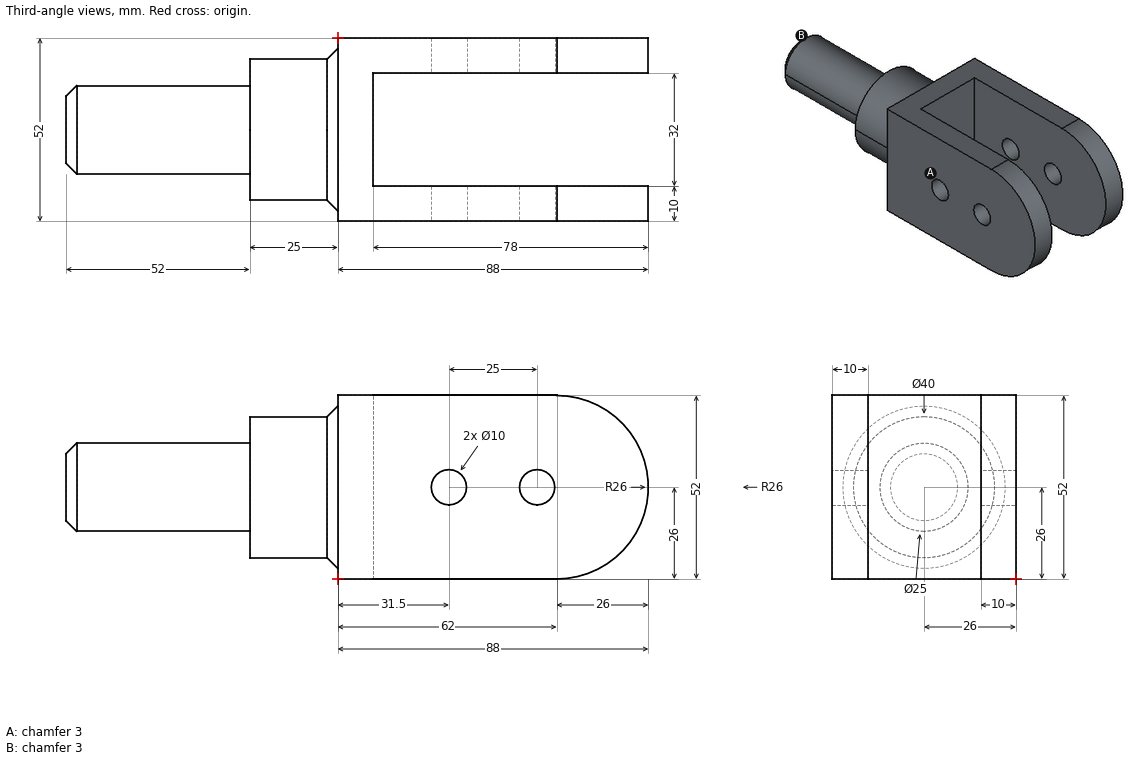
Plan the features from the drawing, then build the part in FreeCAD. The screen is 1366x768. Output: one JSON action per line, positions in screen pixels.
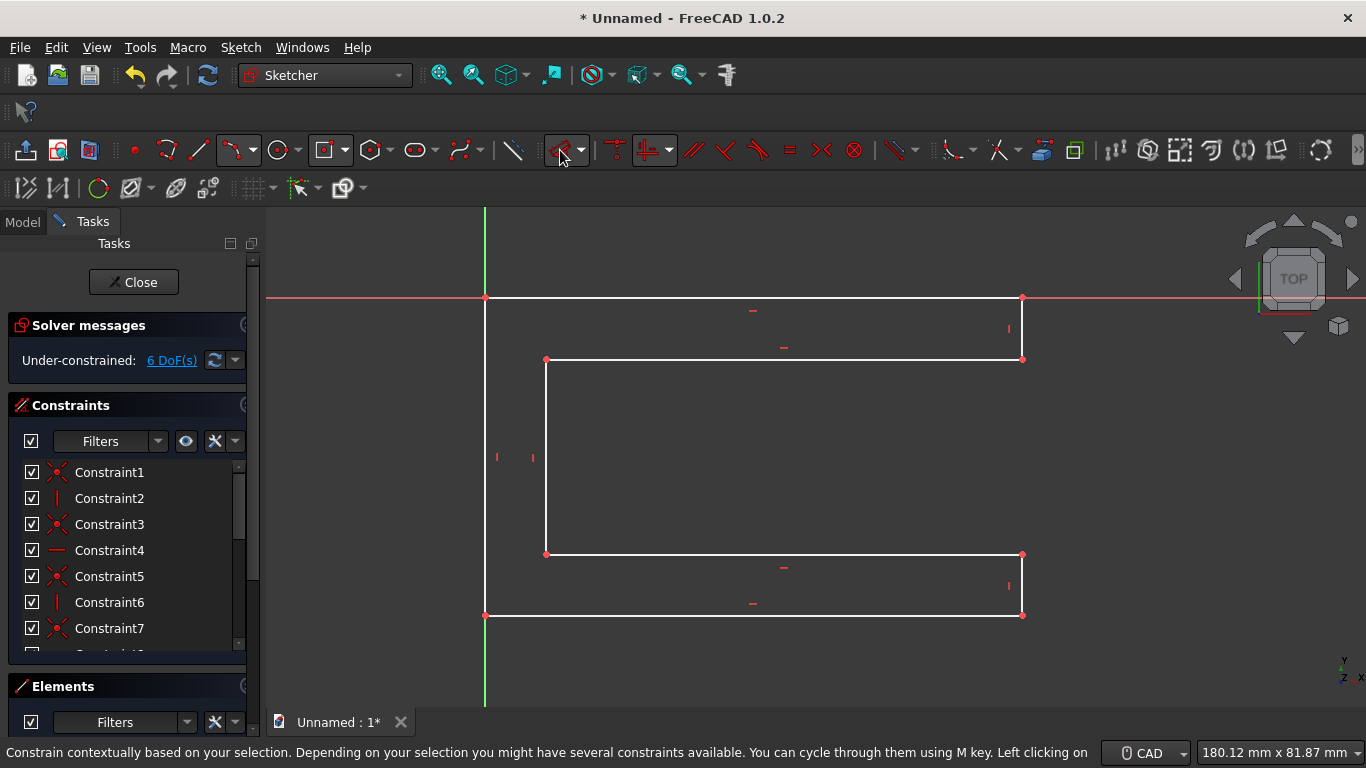
{"action": "left_click", "coordinate": [485, 393]}
{"action": "left_click", "coordinate": [451, 457]}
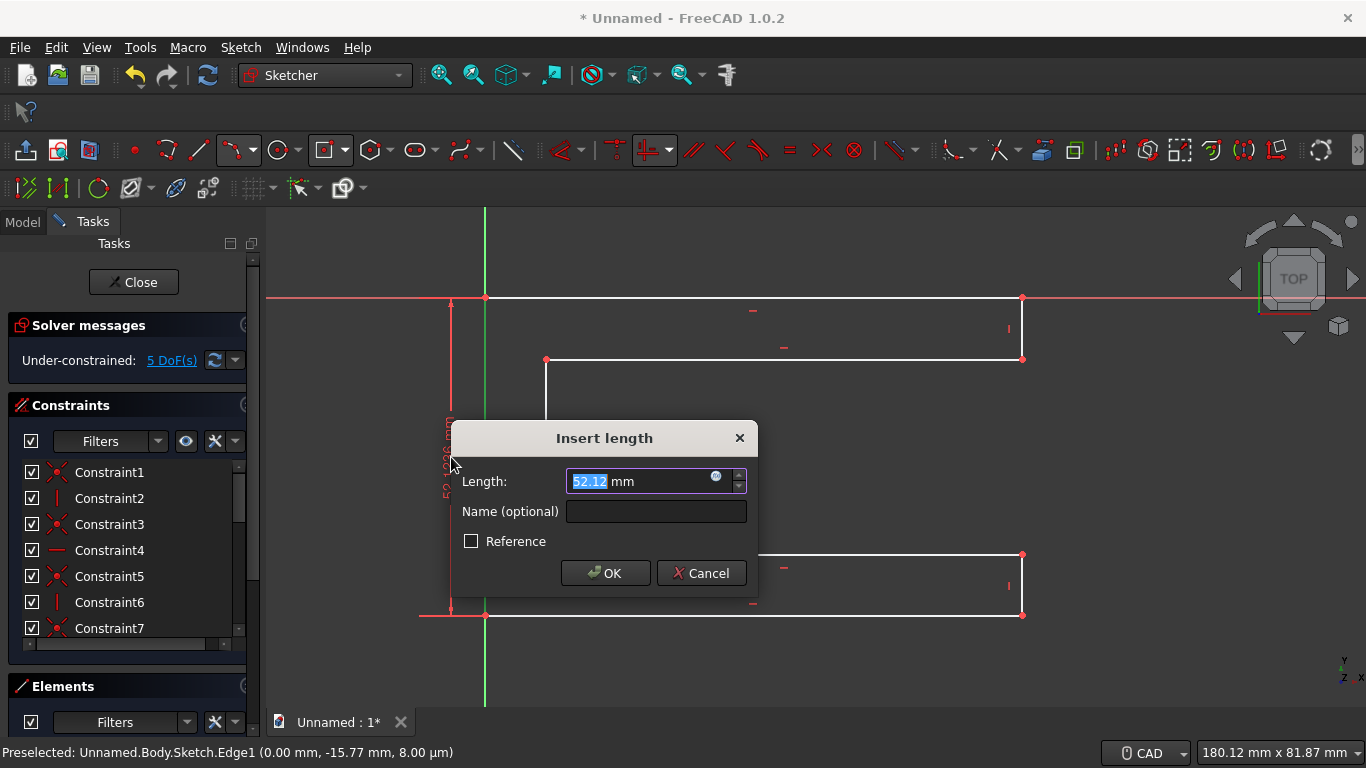
{"action": "type", "text": "52"}
{"action": "key", "text": "Return"}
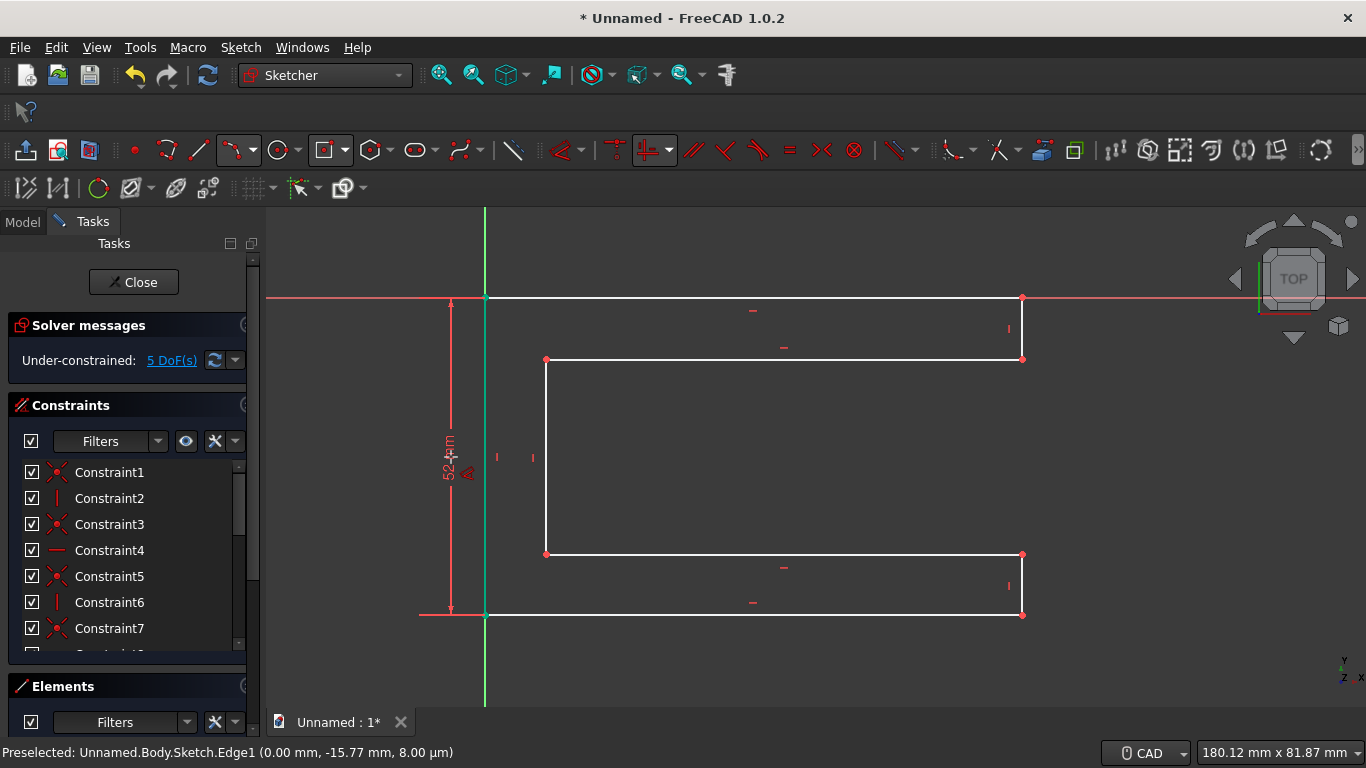
{"action": "left_click", "coordinate": [646, 615]}
{"action": "left_click", "coordinate": [754, 649]}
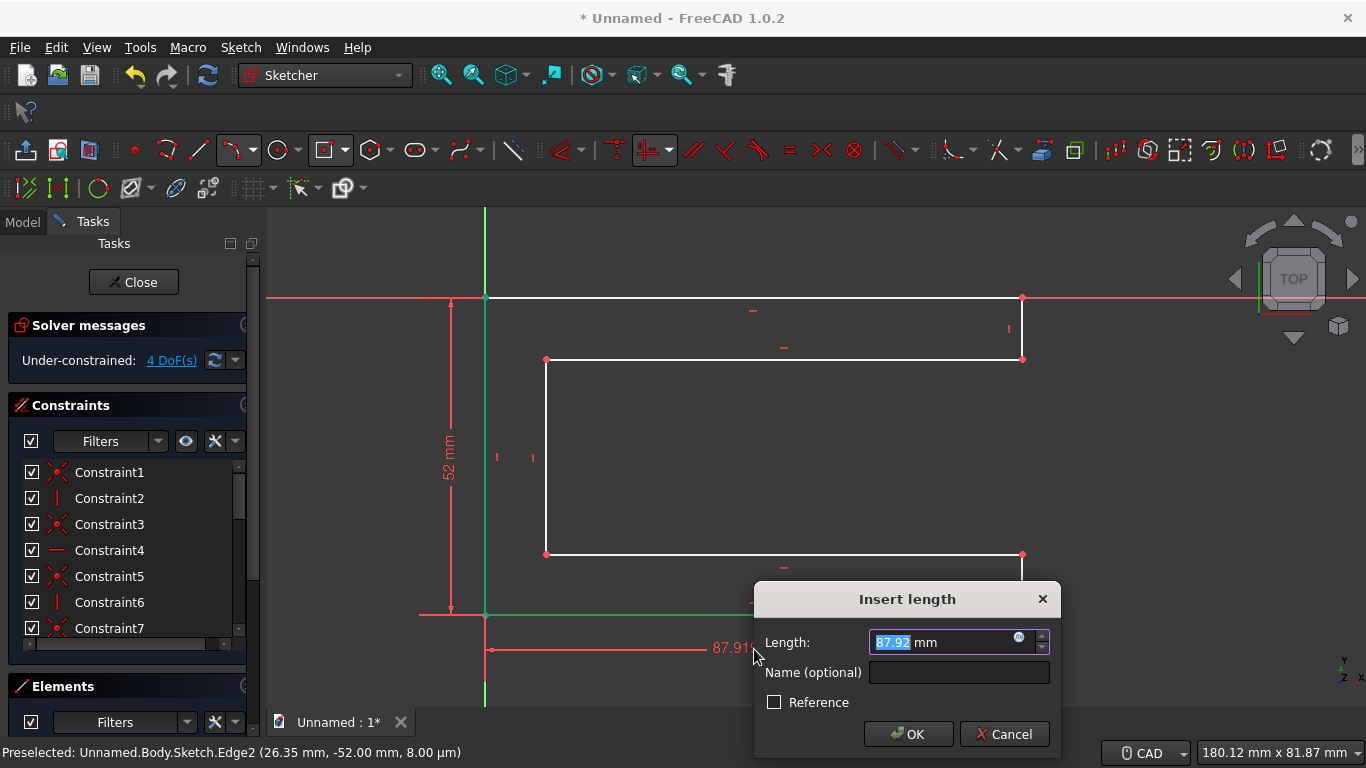
{"action": "type", "text": "88"}
{"action": "key", "text": "Return"}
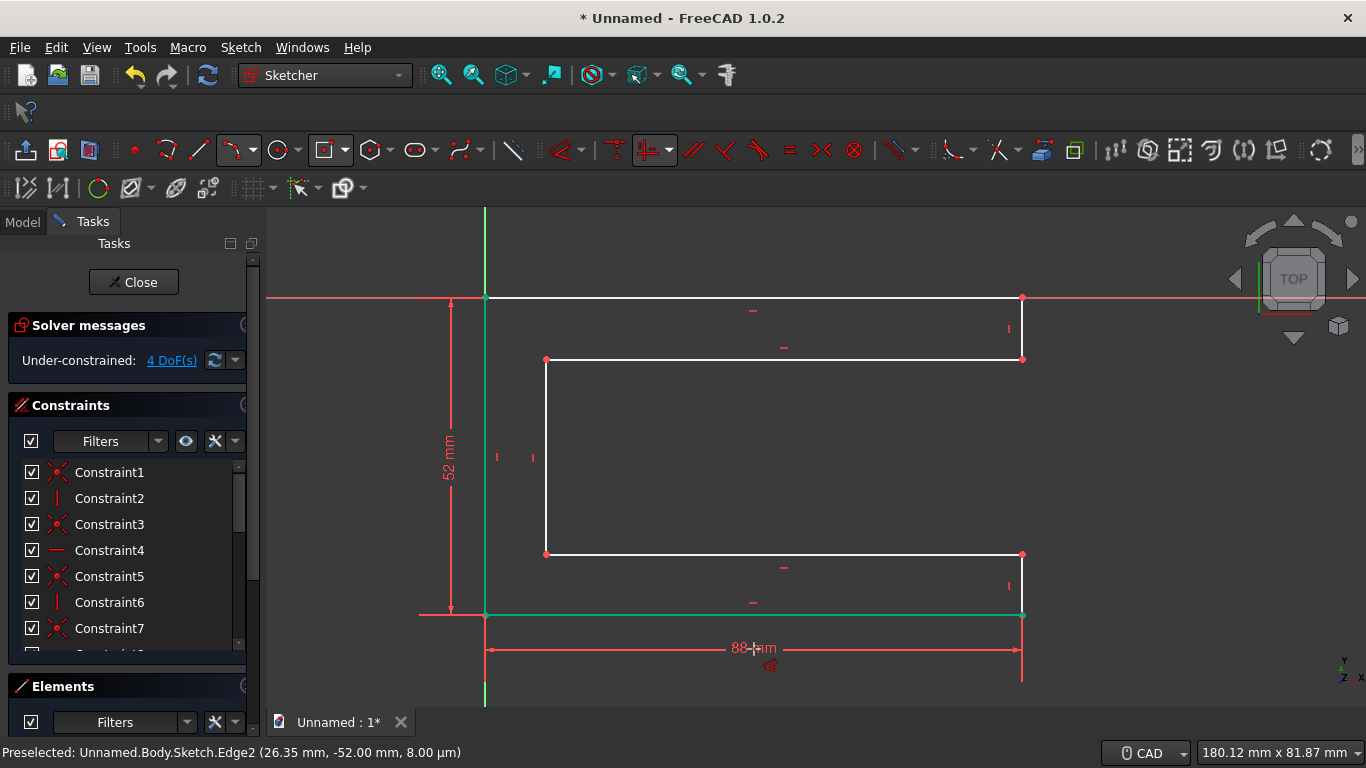
{"action": "left_click", "coordinate": [1022, 597]}
{"action": "left_click", "coordinate": [1056, 585]}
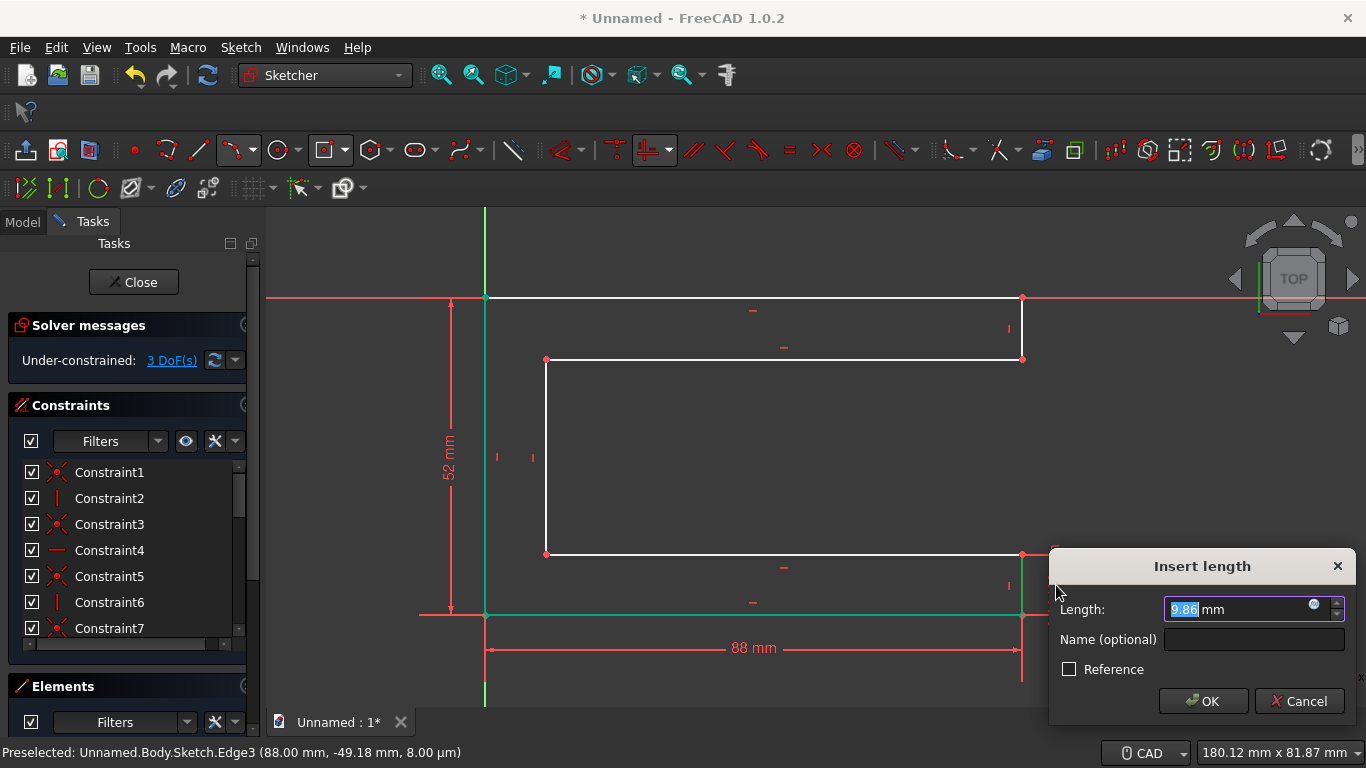
{"action": "type", "text": "10"}
{"action": "key", "text": "Return"}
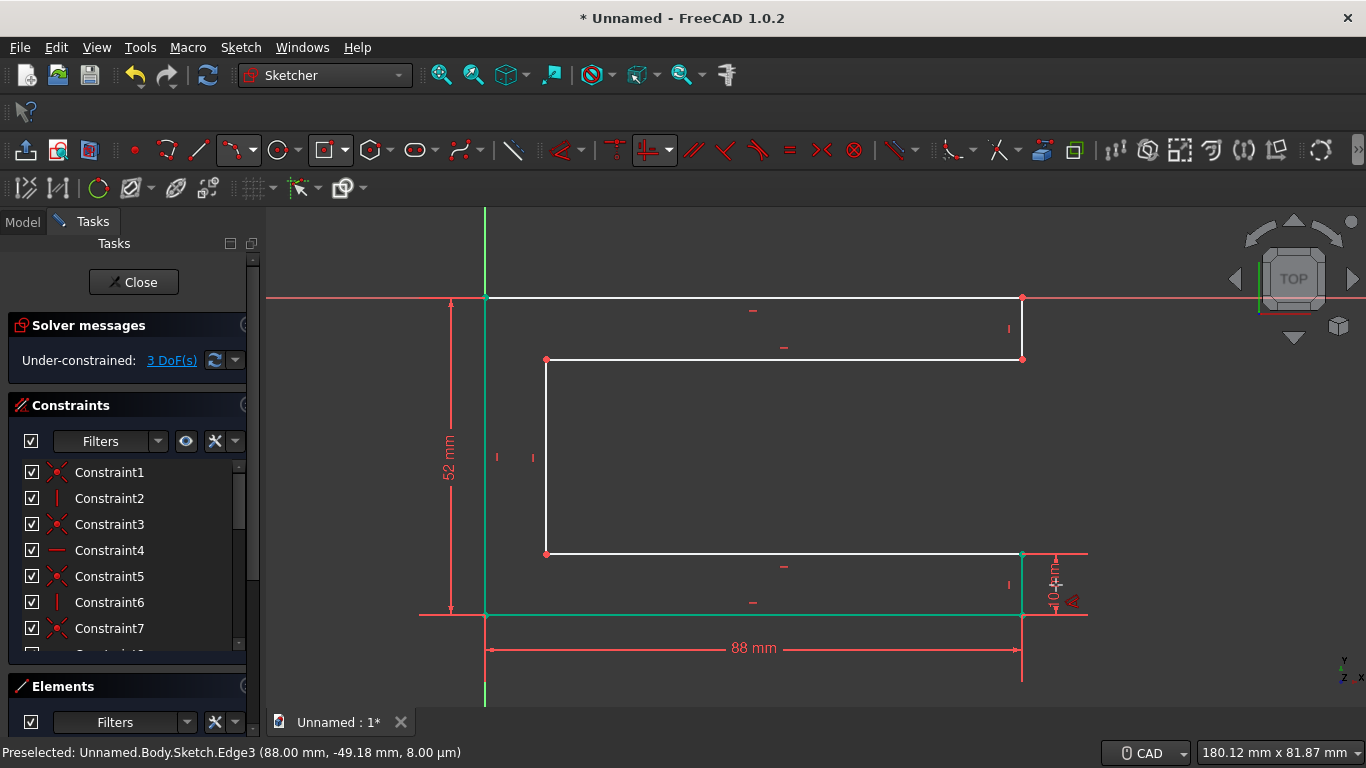
{"action": "left_click", "coordinate": [880, 554]}
{"action": "left_click", "coordinate": [784, 588]}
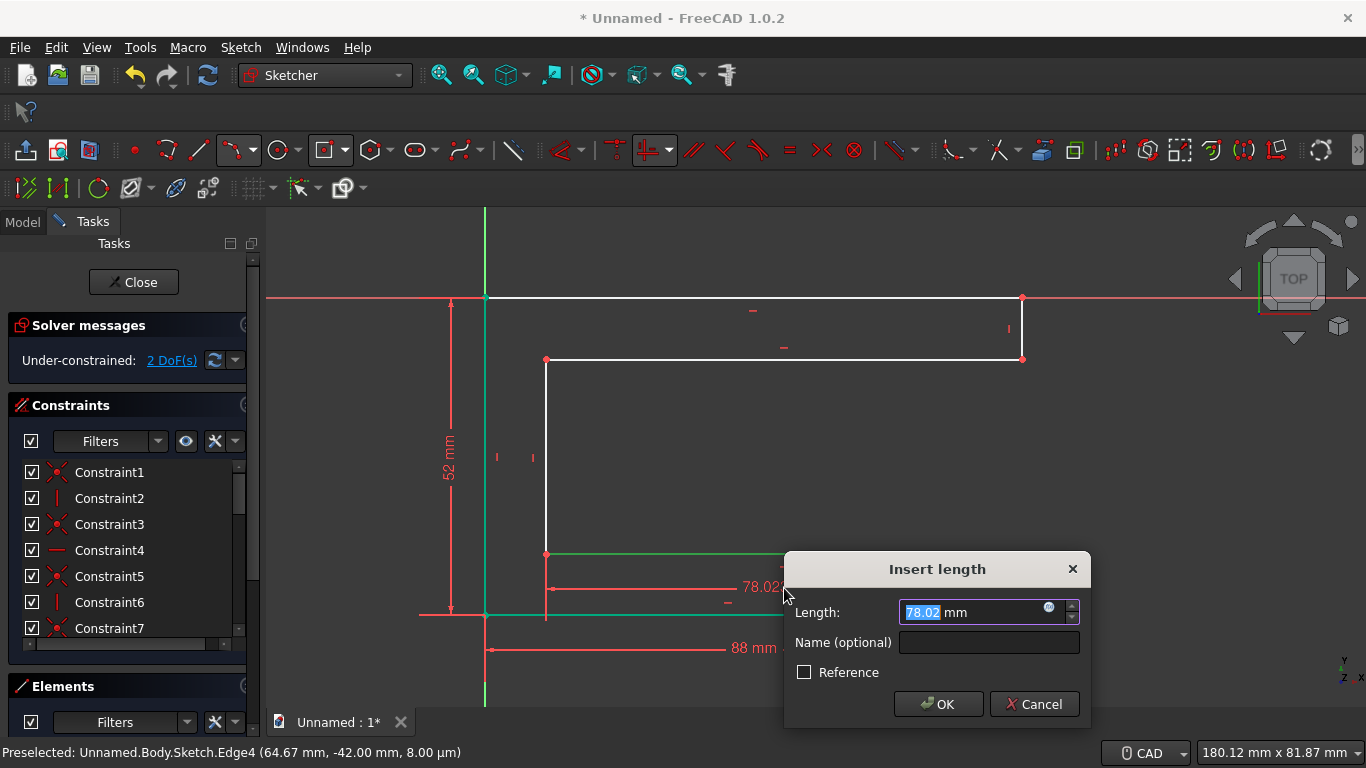
{"action": "type", "text": "78"}
{"action": "key", "text": "Return"}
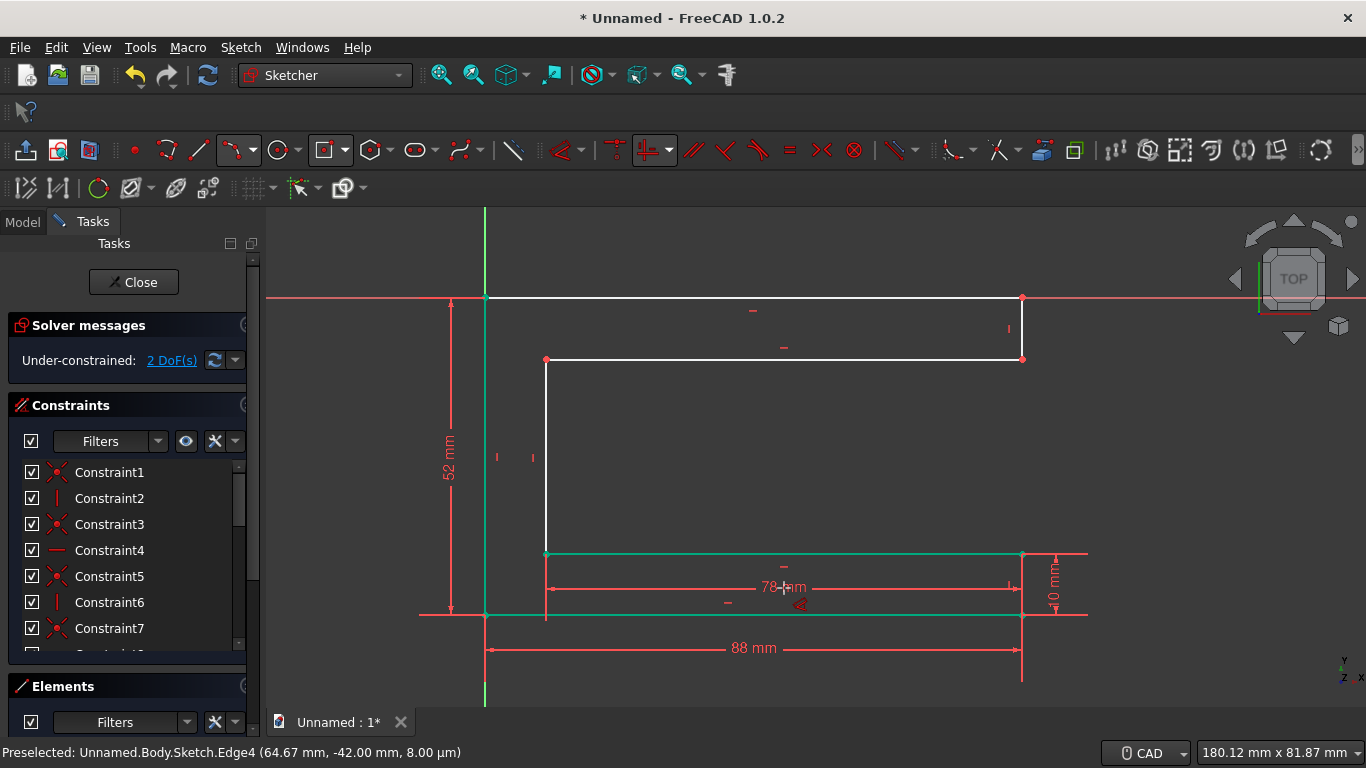
{"action": "left_click", "coordinate": [546, 496]}
{"action": "left_click", "coordinate": [512, 412]}